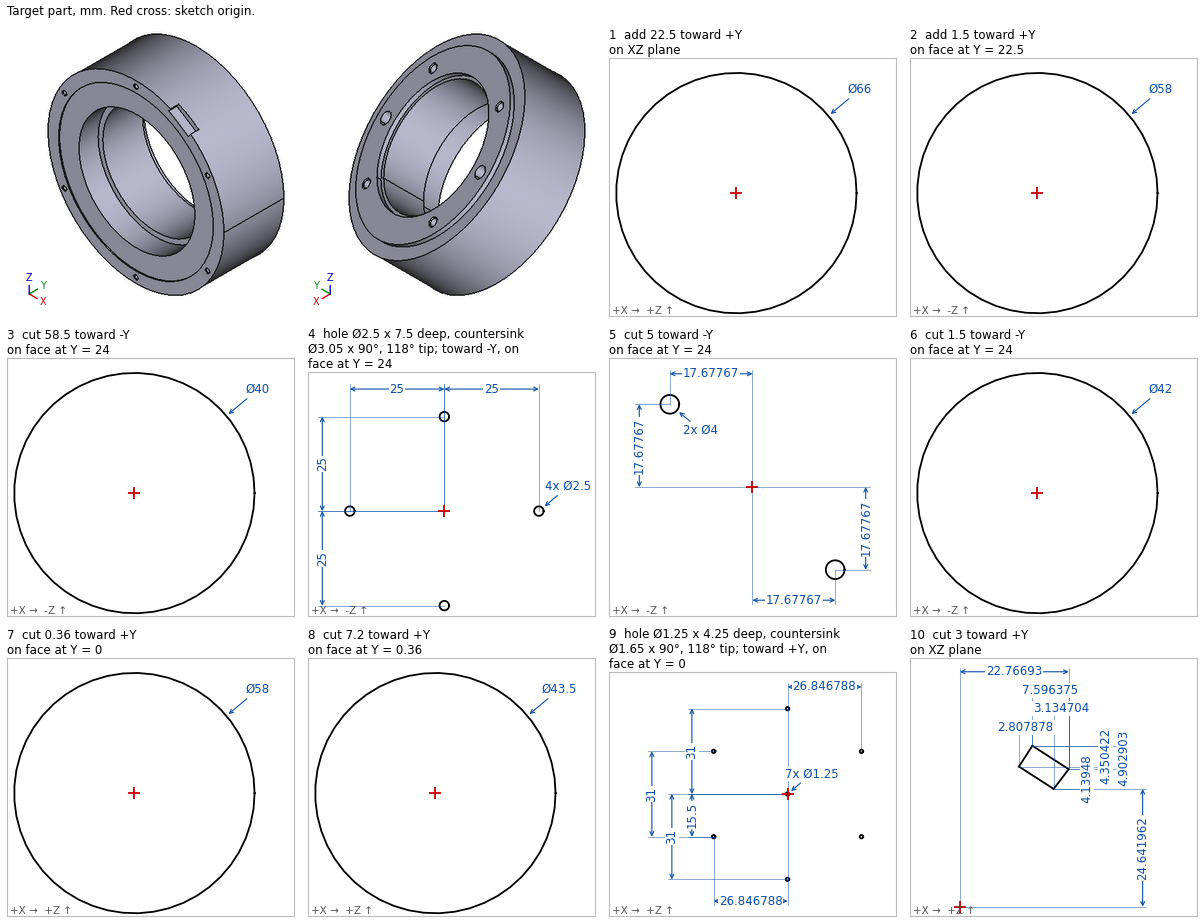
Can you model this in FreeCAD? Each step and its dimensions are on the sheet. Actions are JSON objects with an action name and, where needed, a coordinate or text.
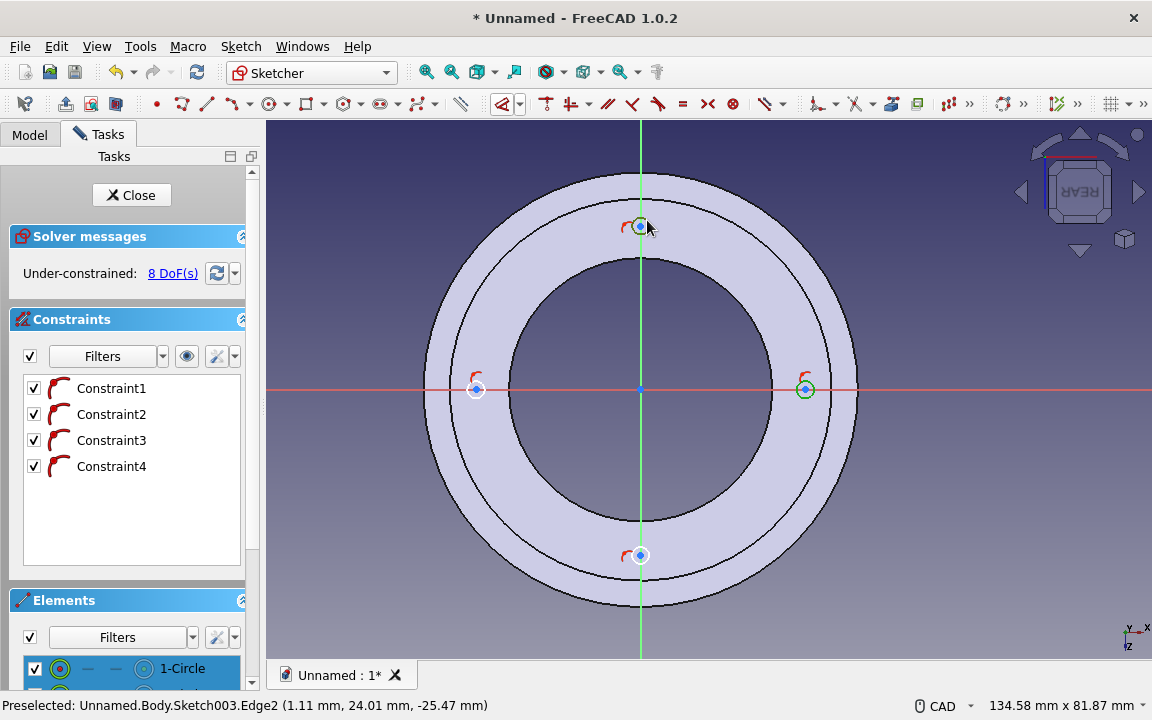
{"action": "scroll", "coordinate": [482, 384], "scroll_direction": "up", "scroll_amount": 5}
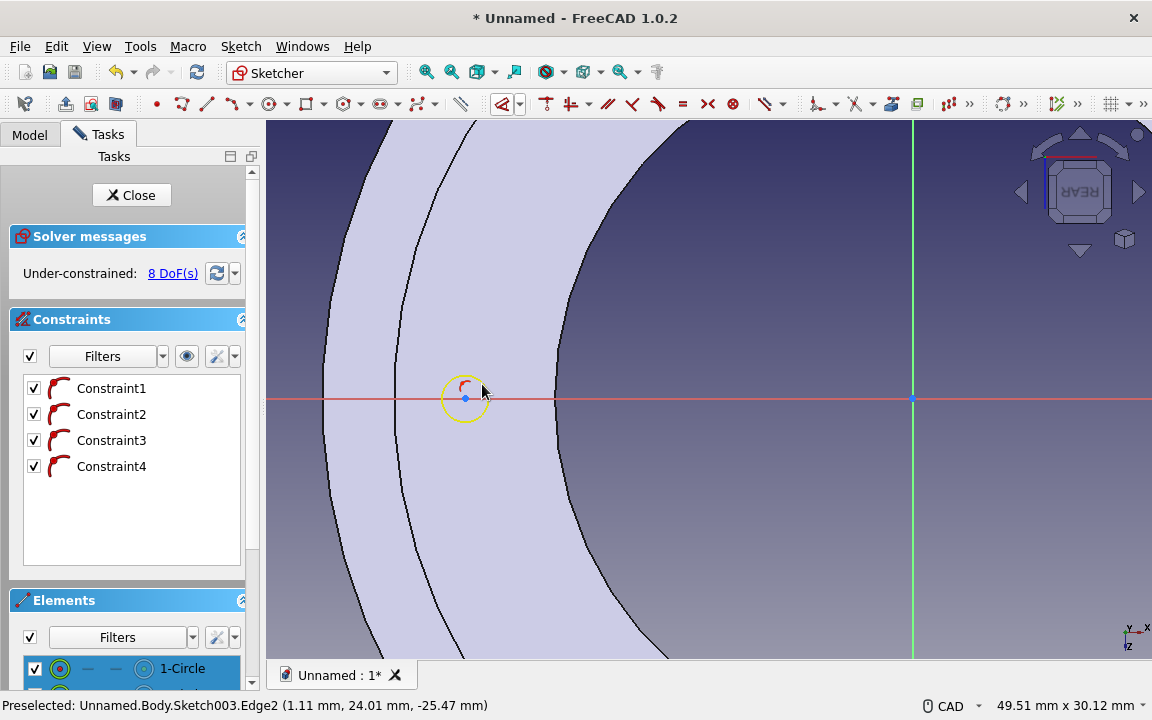
{"action": "left_click", "coordinate": [482, 382]}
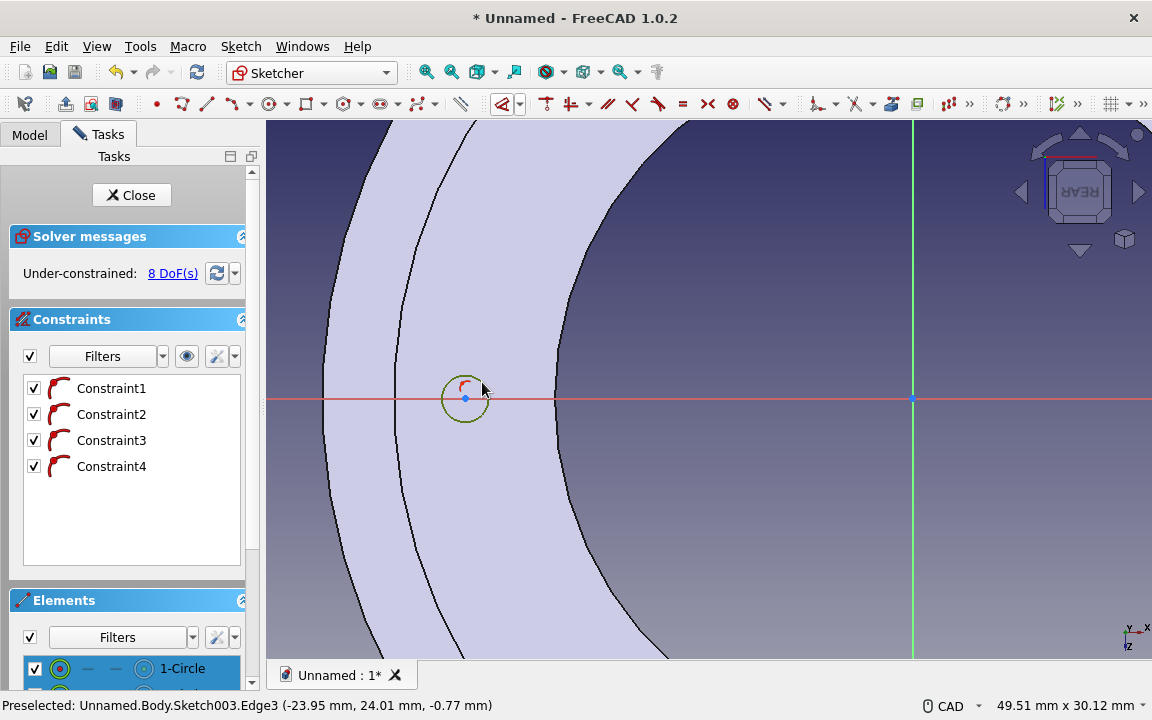
{"action": "scroll", "coordinate": [482, 384], "scroll_direction": "down", "scroll_amount": 5}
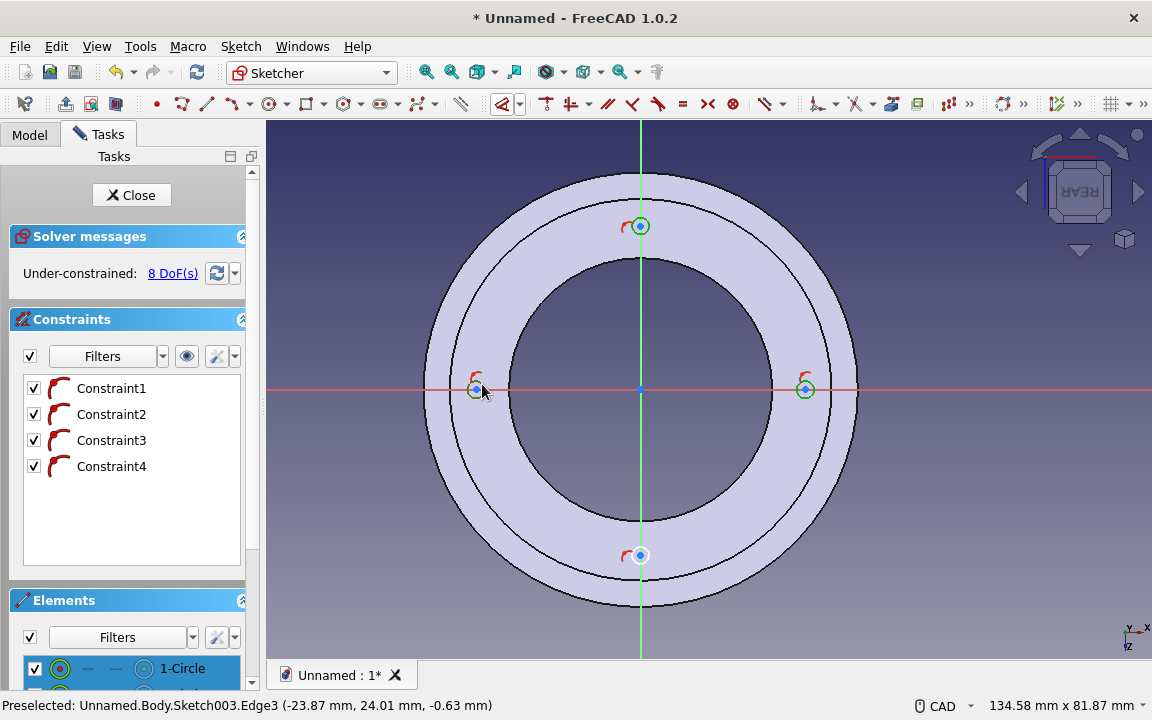
{"action": "scroll", "coordinate": [647, 549], "scroll_direction": "up", "scroll_amount": 5}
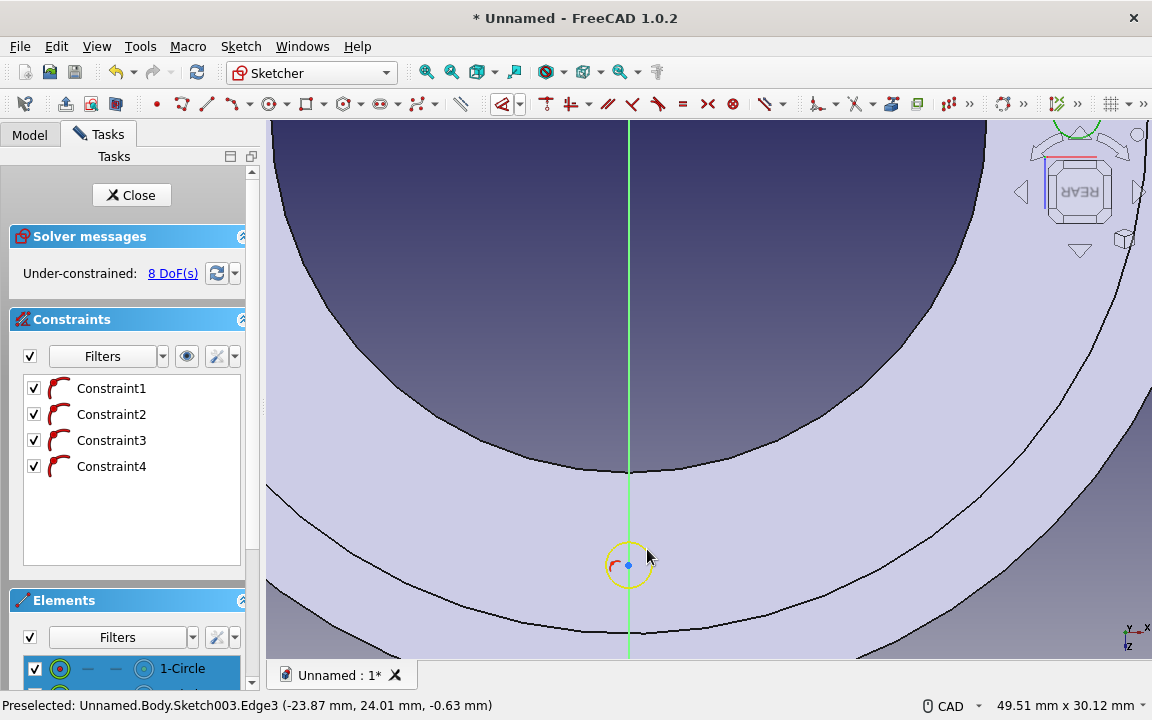
{"action": "left_click", "coordinate": [645, 549]}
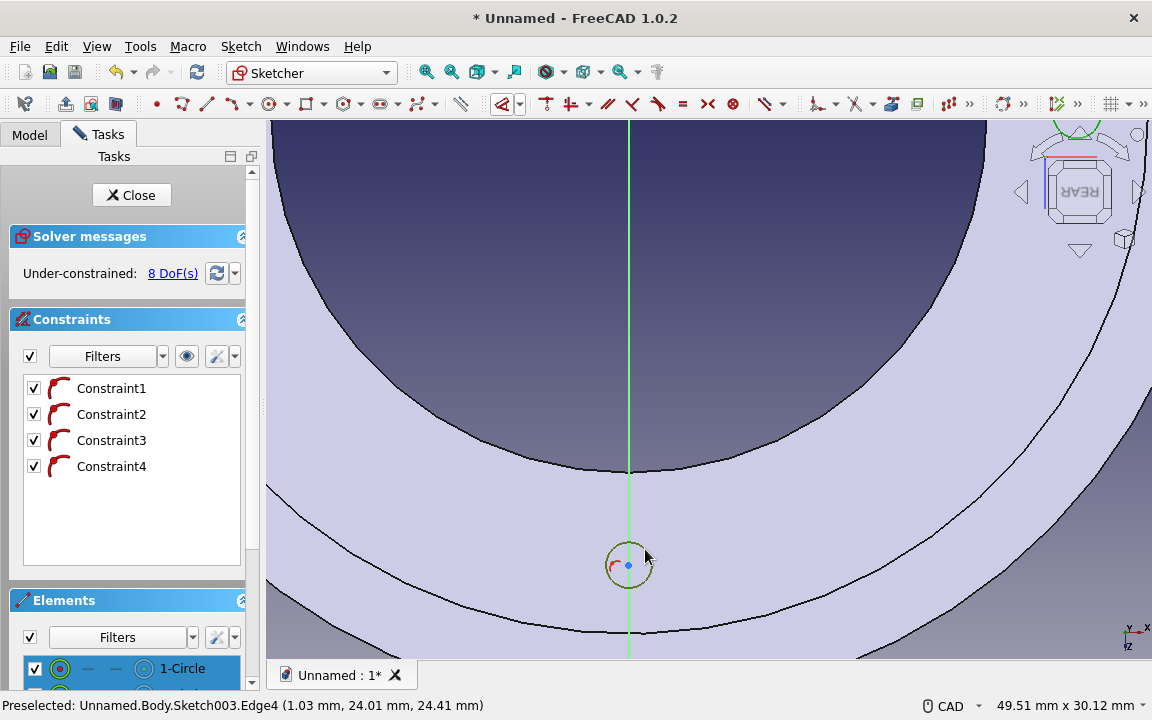
{"action": "left_click", "coordinate": [683, 104]}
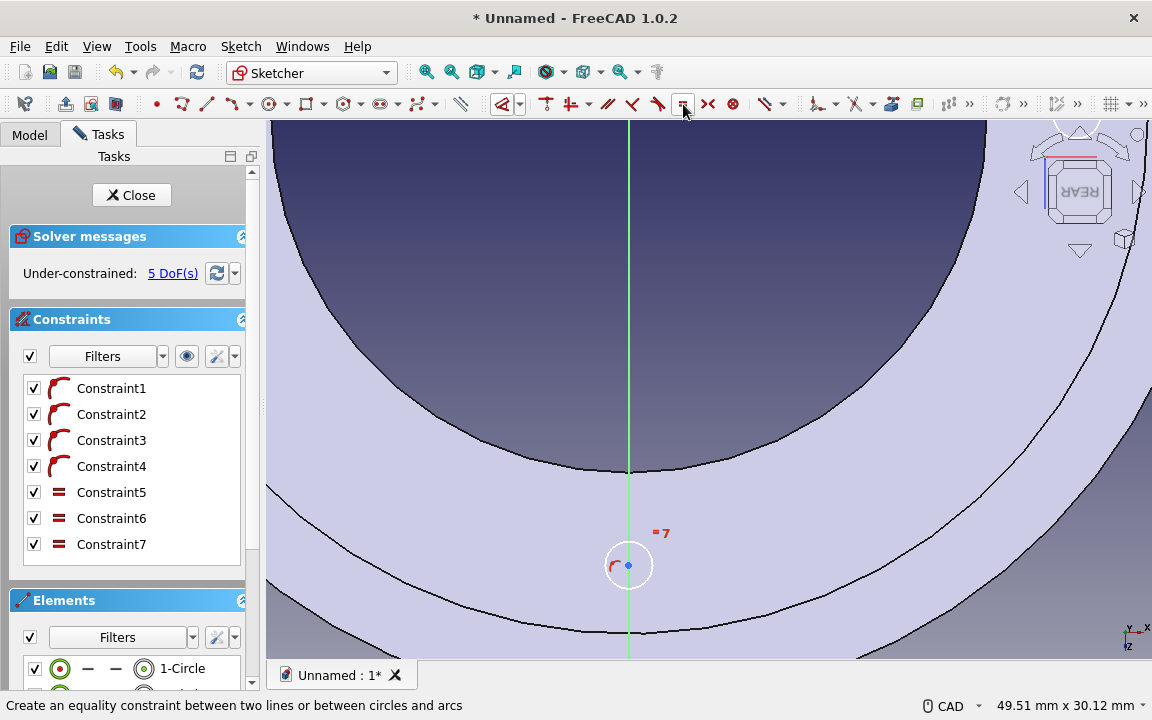
{"action": "scroll", "coordinate": [647, 549], "scroll_direction": "down", "scroll_amount": 5}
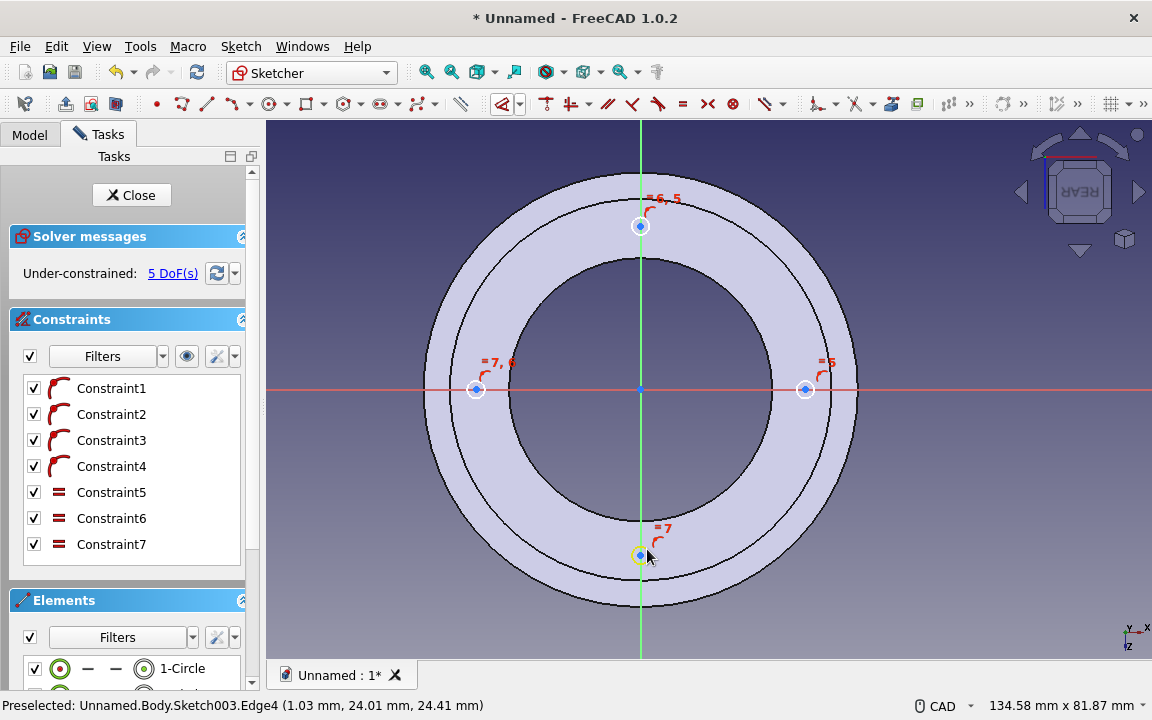
{"action": "scroll", "coordinate": [812, 384], "scroll_direction": "up", "scroll_amount": 5}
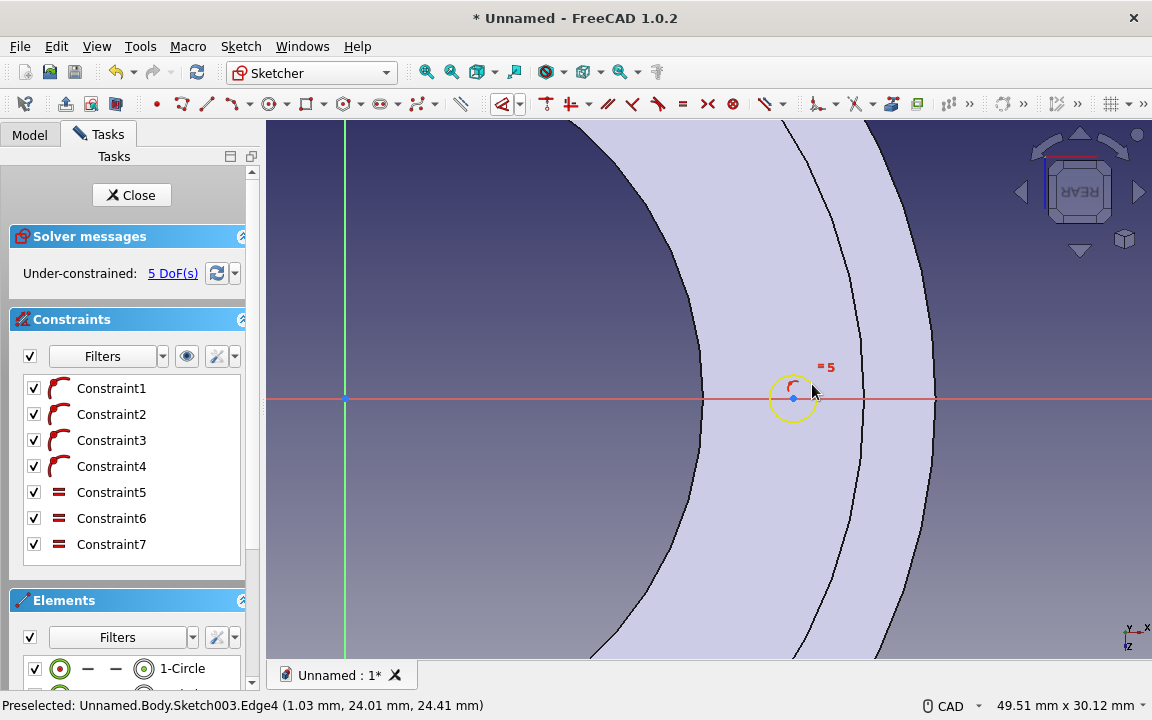
{"action": "left_click", "coordinate": [810, 382]}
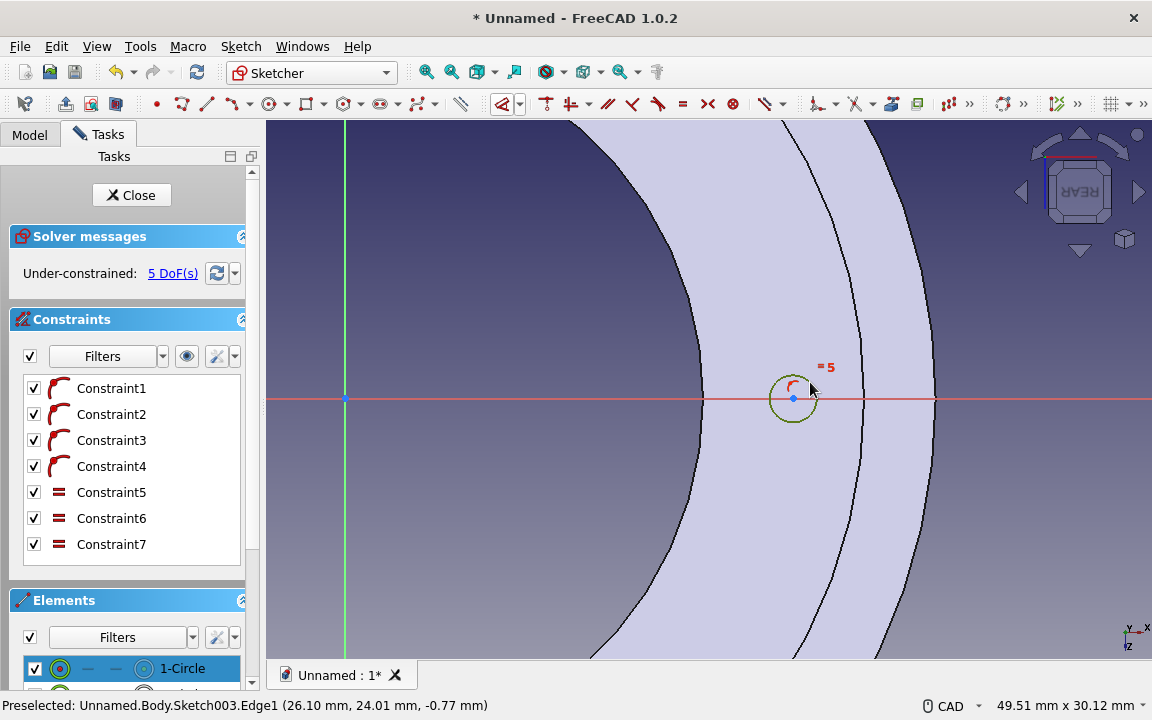
{"action": "left_click", "coordinate": [520, 104]}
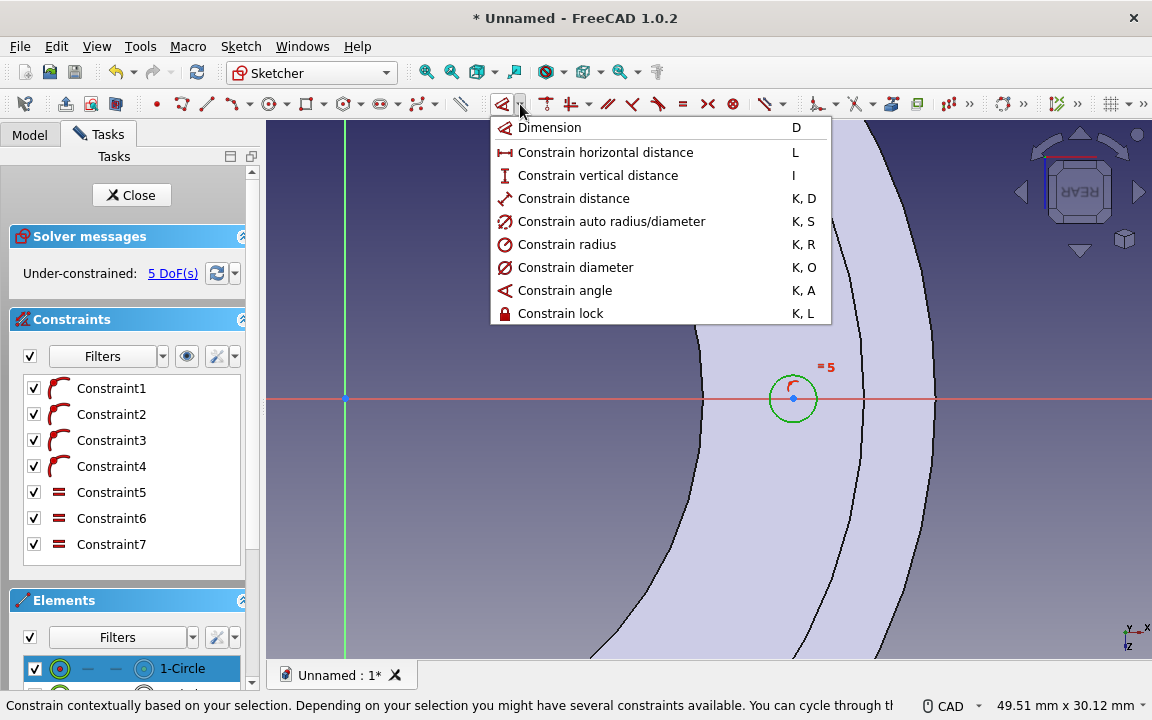
{"action": "left_click", "coordinate": [661, 268]}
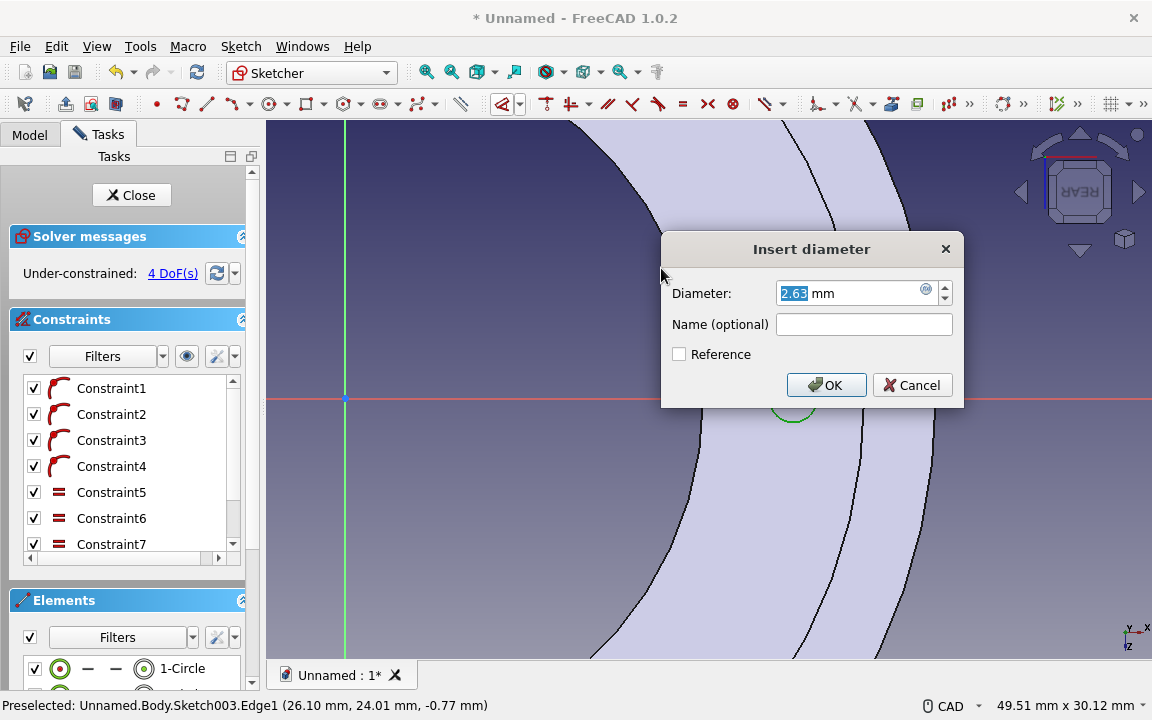
{"action": "type", "text": "2.5"}
{"action": "key", "text": "Return"}